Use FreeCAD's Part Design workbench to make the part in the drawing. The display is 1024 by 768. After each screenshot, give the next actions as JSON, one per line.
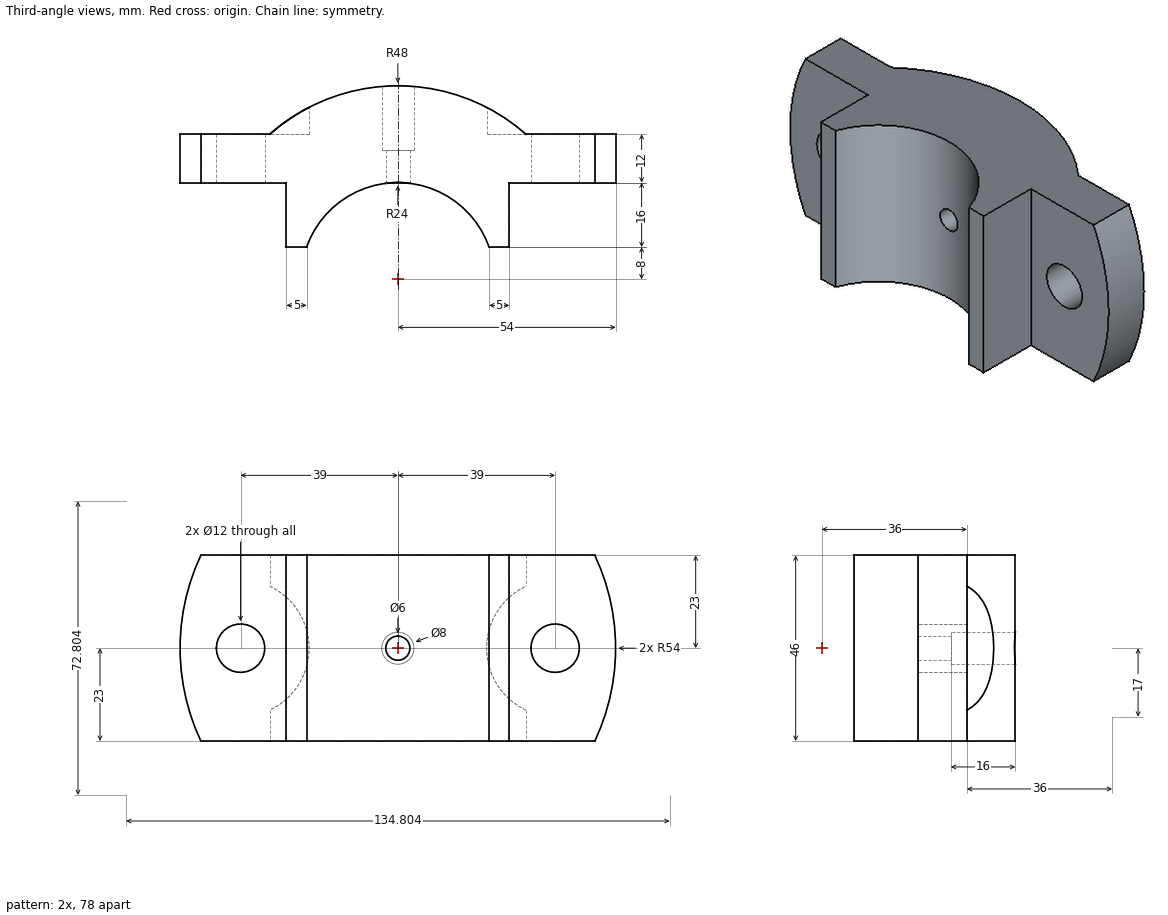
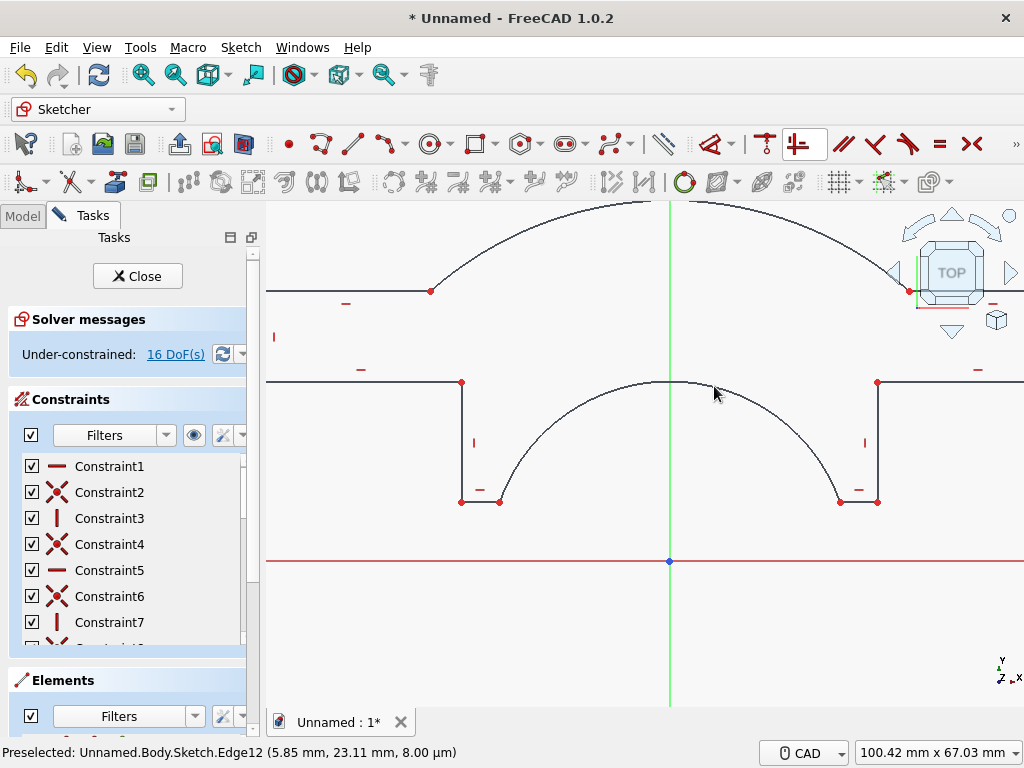
{"action": "left_click", "coordinate": [822, 234]}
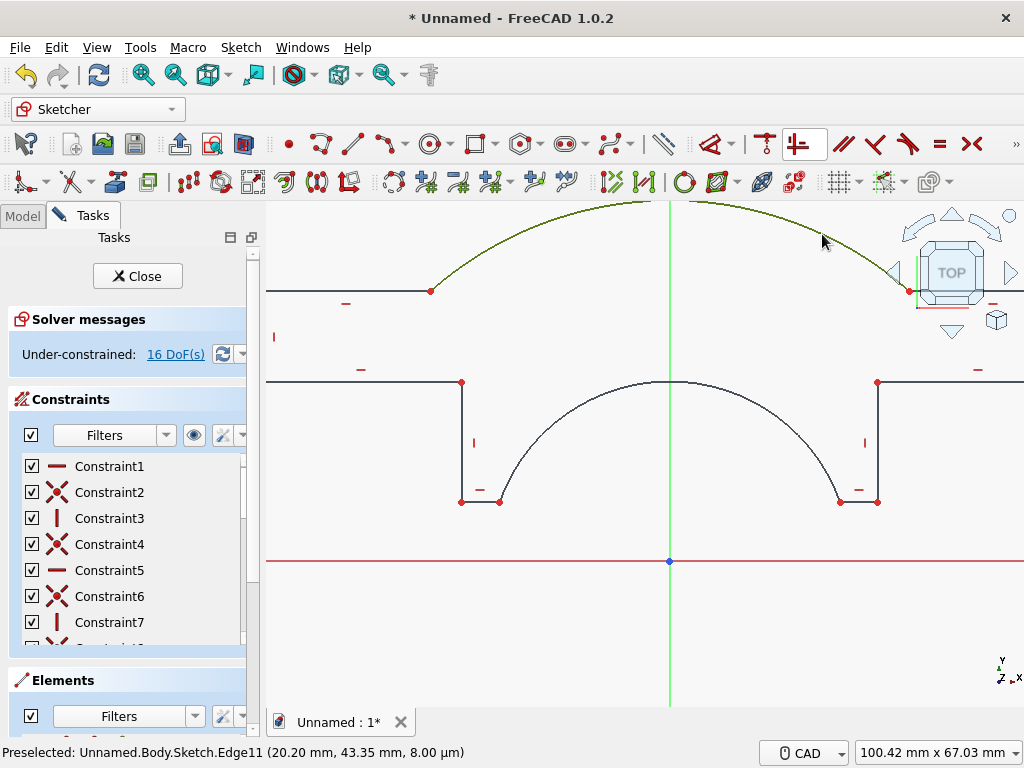
{"action": "left_click", "coordinate": [755, 403]}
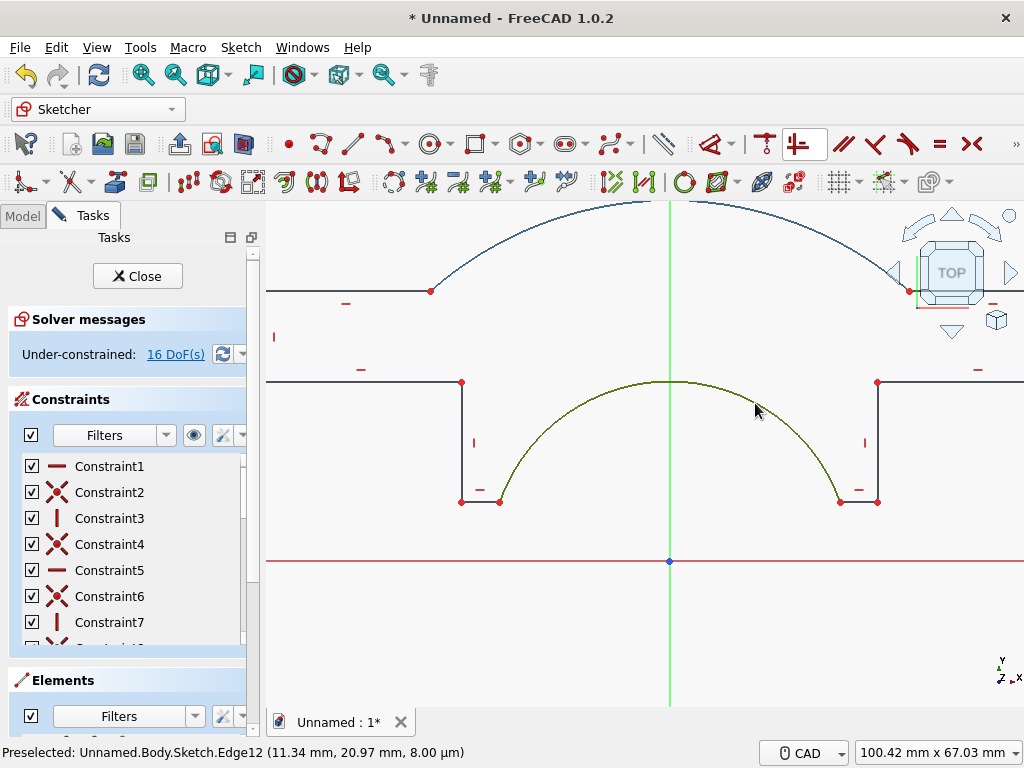
{"action": "key", "text": "c"}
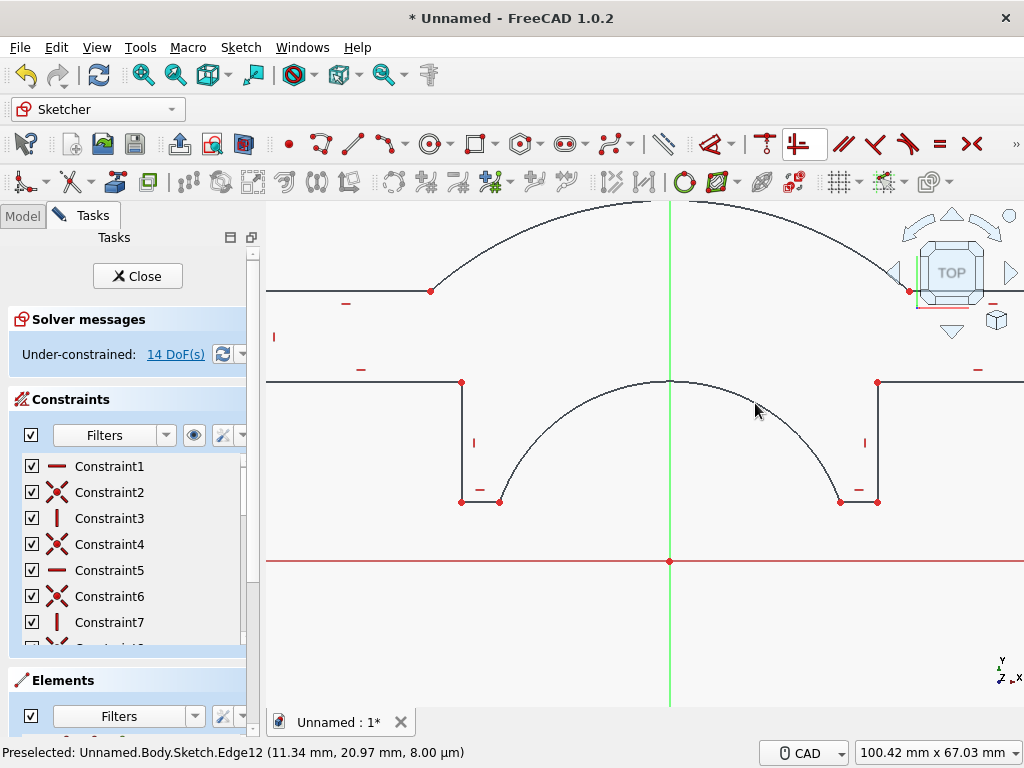
{"action": "left_click_drag", "start_coordinate": [660, 551], "coordinate": [680, 572]}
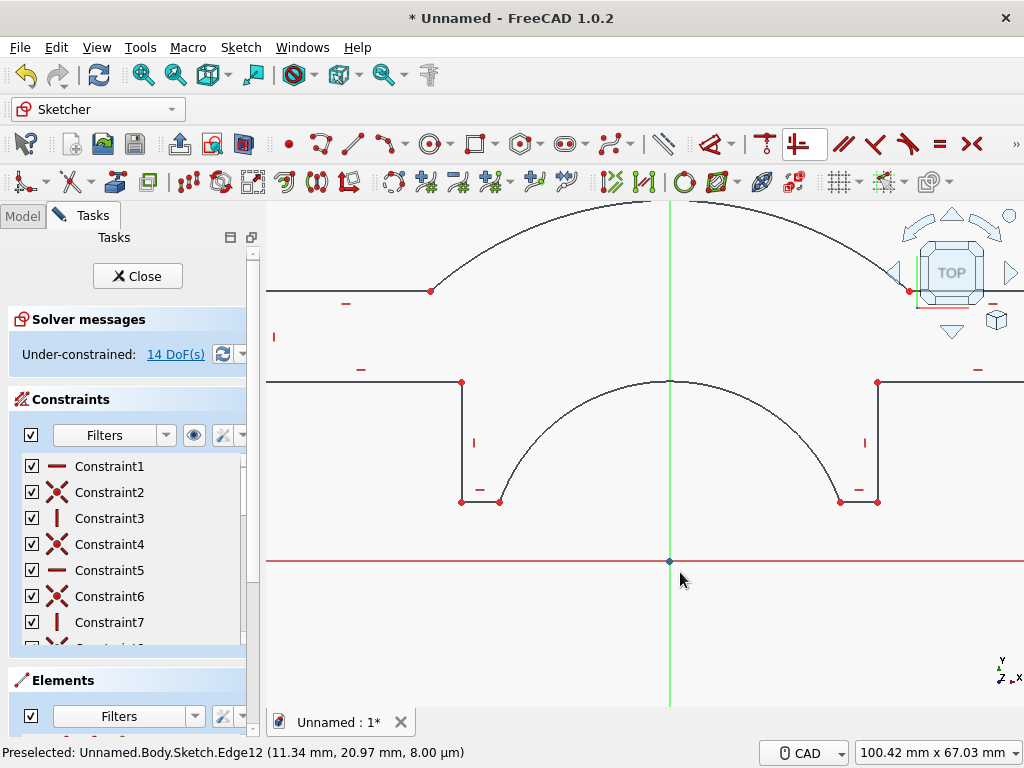
{"action": "left_click", "coordinate": [766, 144]}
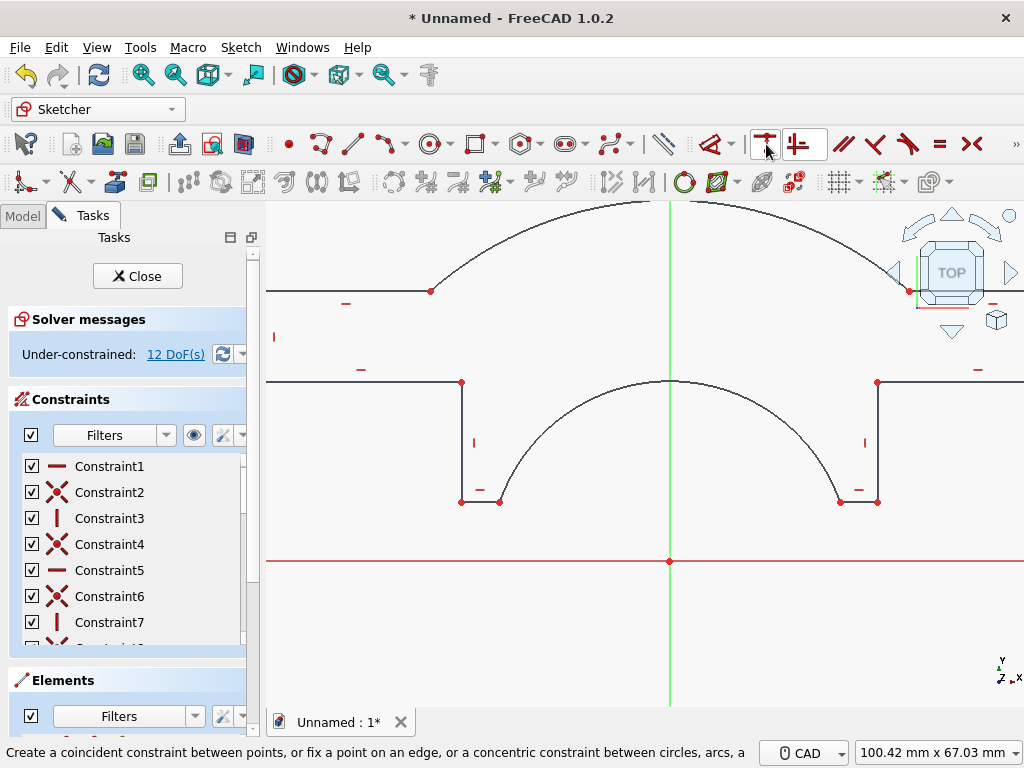
{"action": "scroll", "coordinate": [500, 514], "scroll_direction": "down", "scroll_amount": 4}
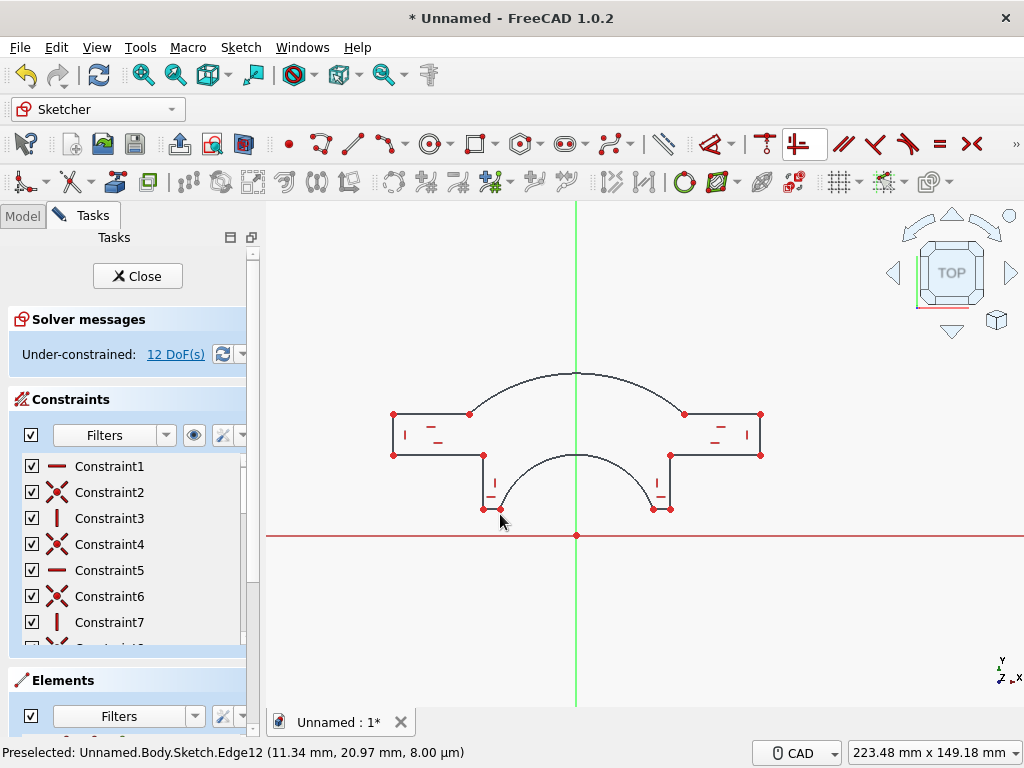
{"action": "left_click", "coordinate": [760, 414]}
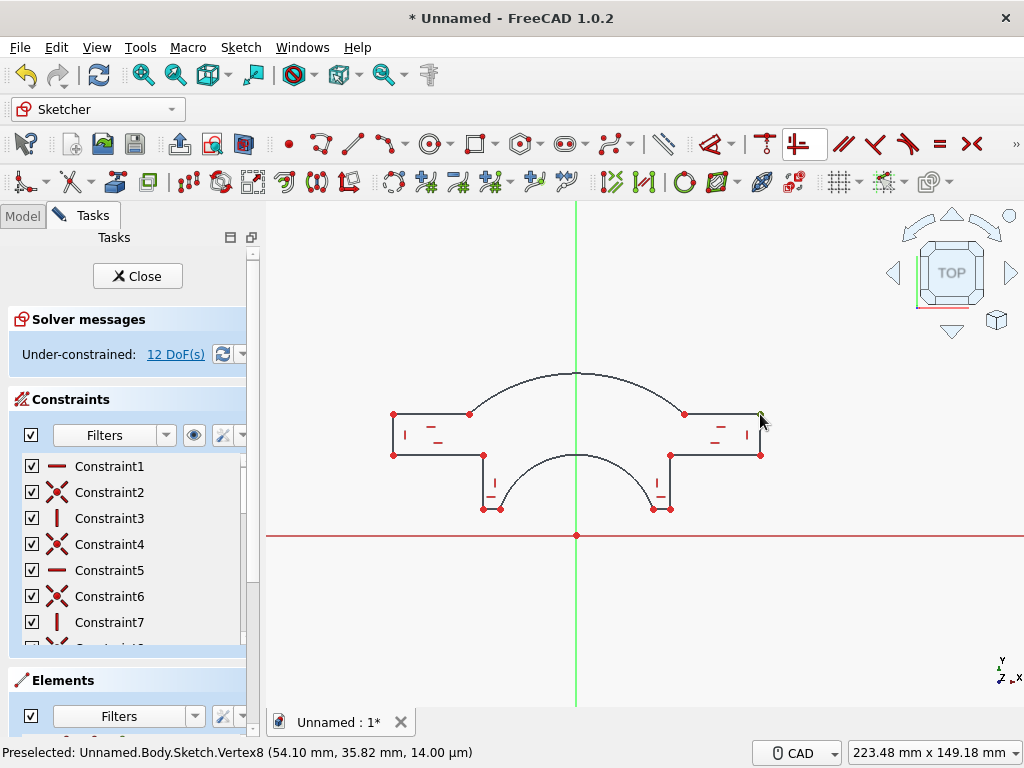
{"action": "left_click", "coordinate": [393, 414]}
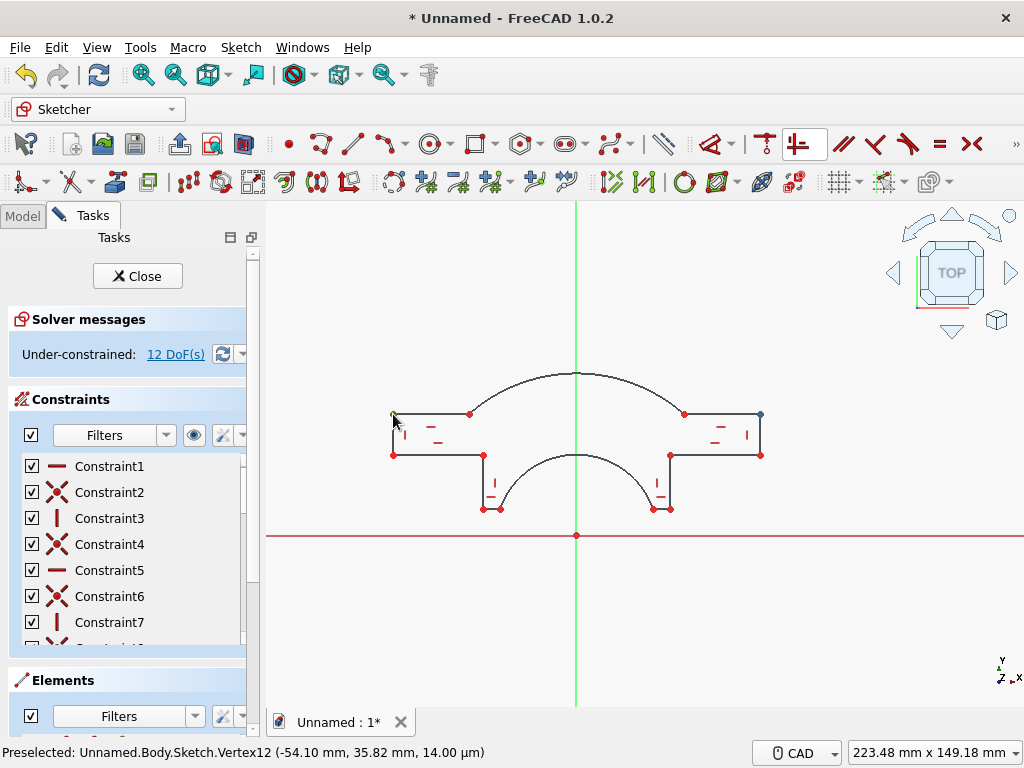
{"action": "left_click", "coordinate": [577, 647]}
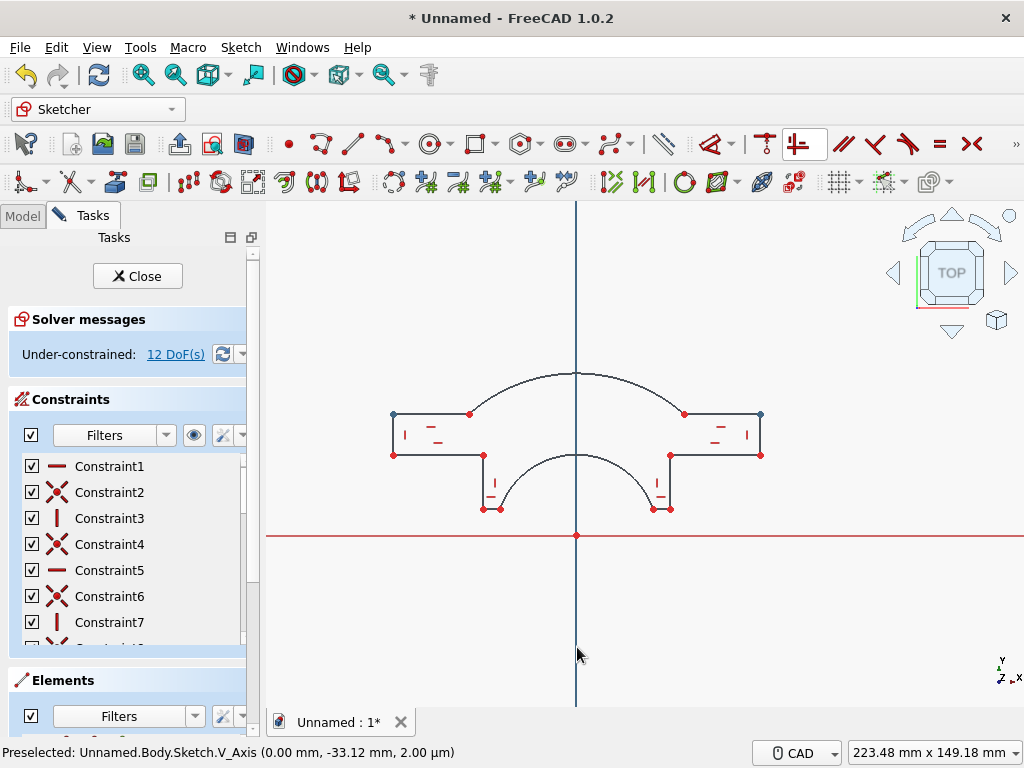
{"action": "left_click", "coordinate": [972, 144]}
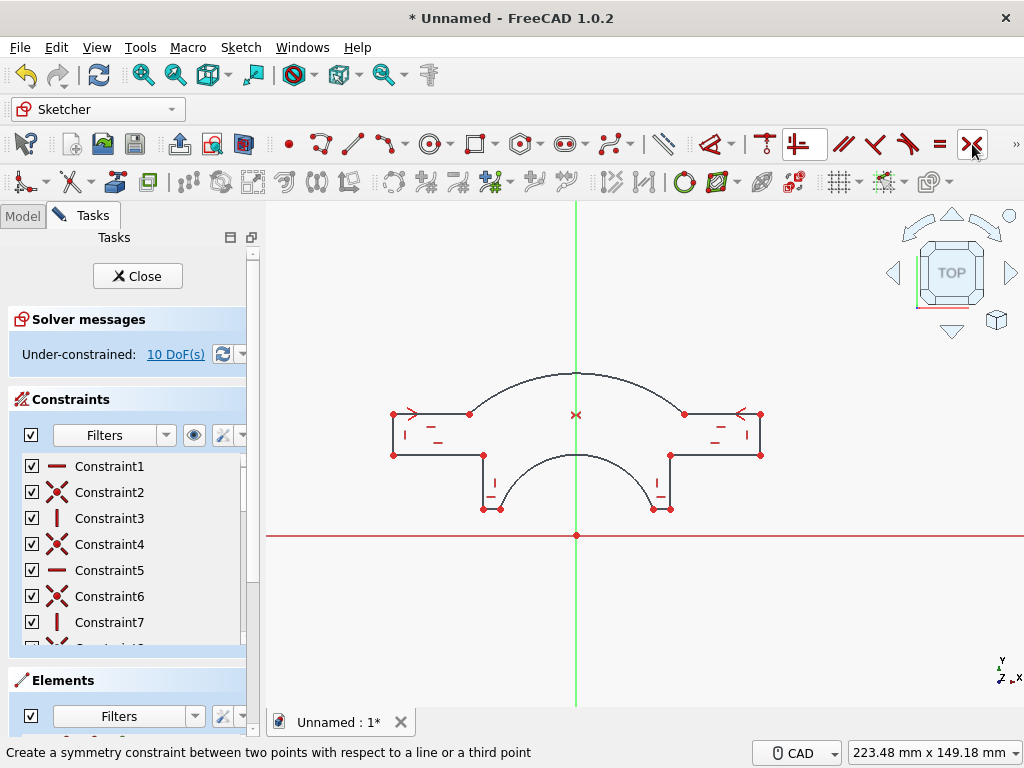
{"action": "left_click", "coordinate": [670, 455]}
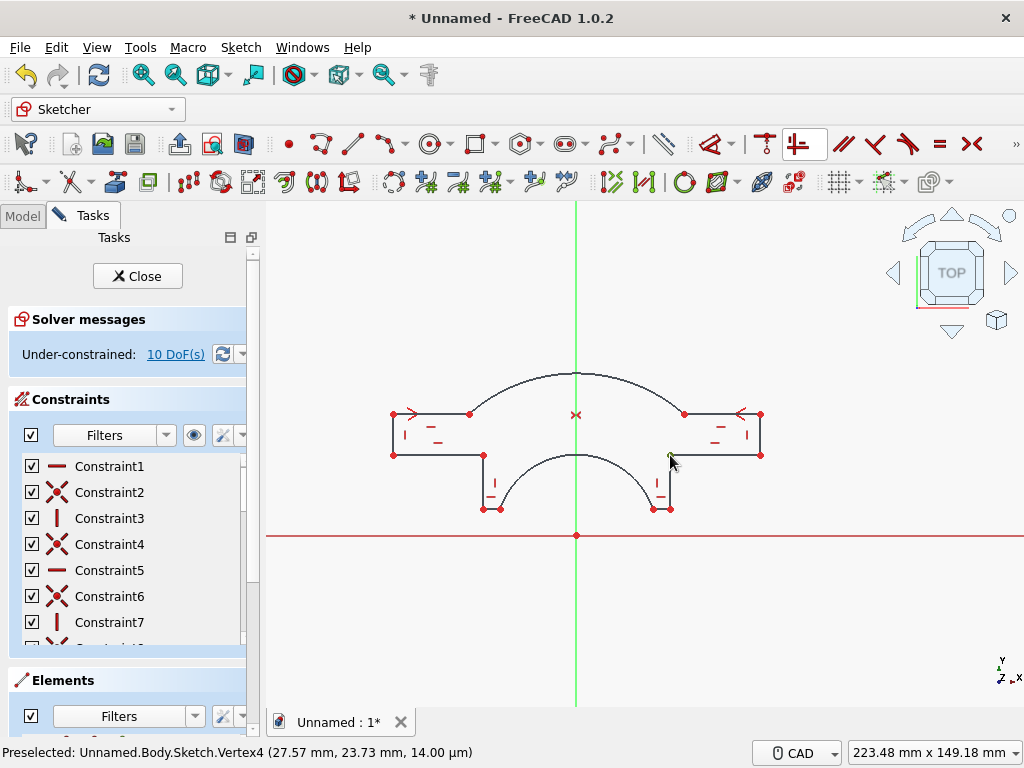
{"action": "left_click", "coordinate": [483, 455]}